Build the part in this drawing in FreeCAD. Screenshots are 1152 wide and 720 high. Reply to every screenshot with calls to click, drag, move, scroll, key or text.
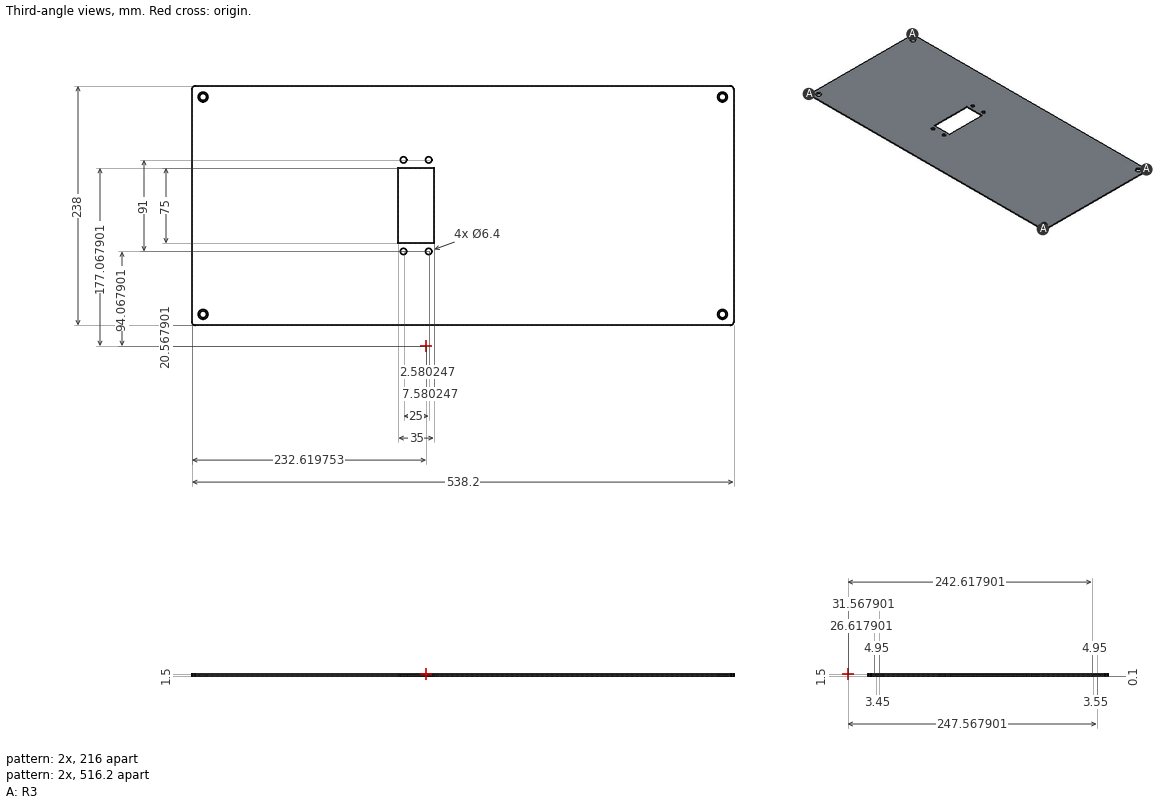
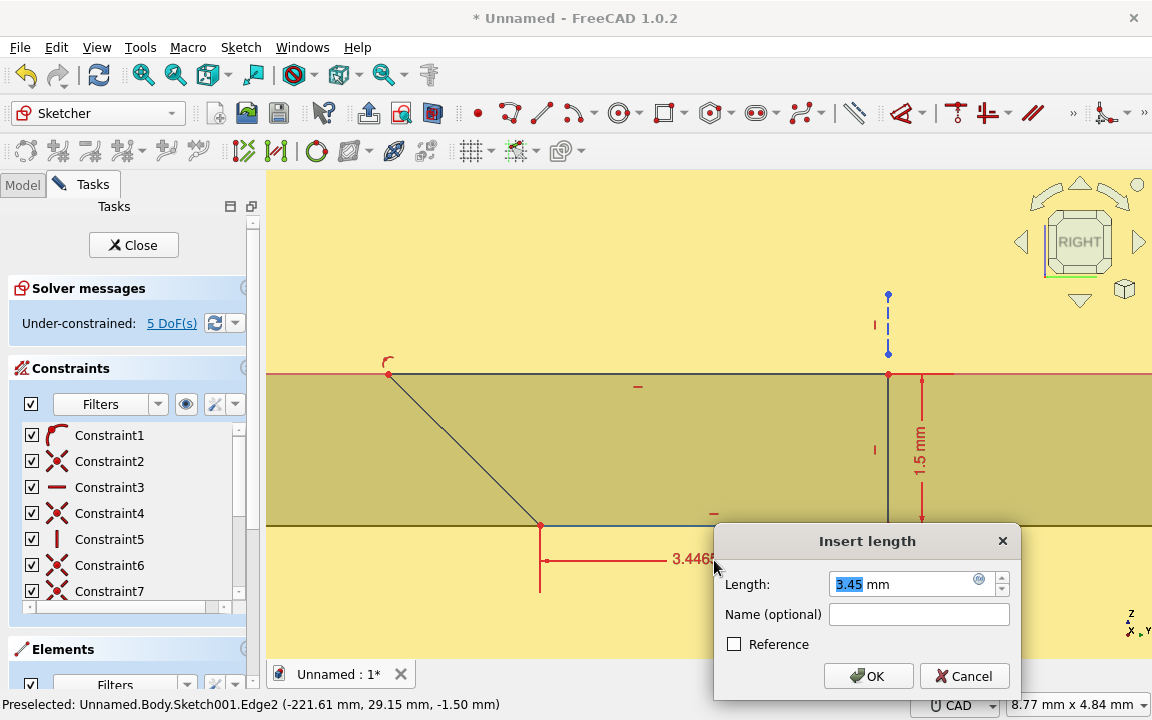
text(3.45)
key(Return)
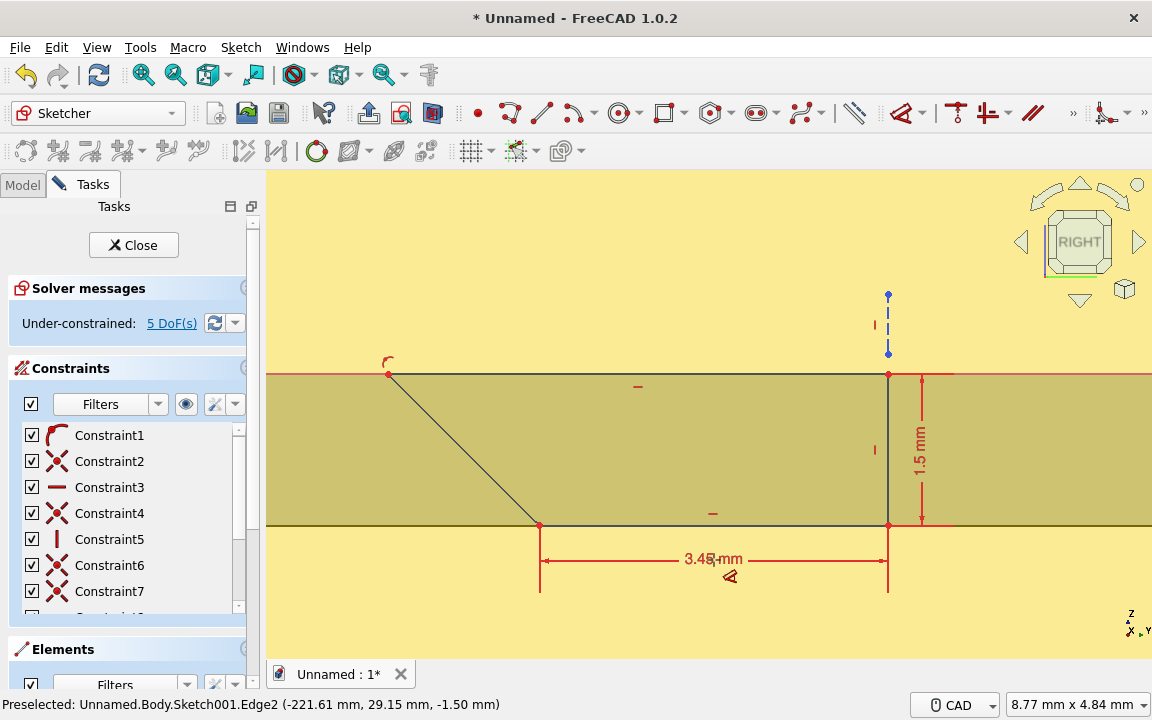
click(738, 374)
click(638, 340)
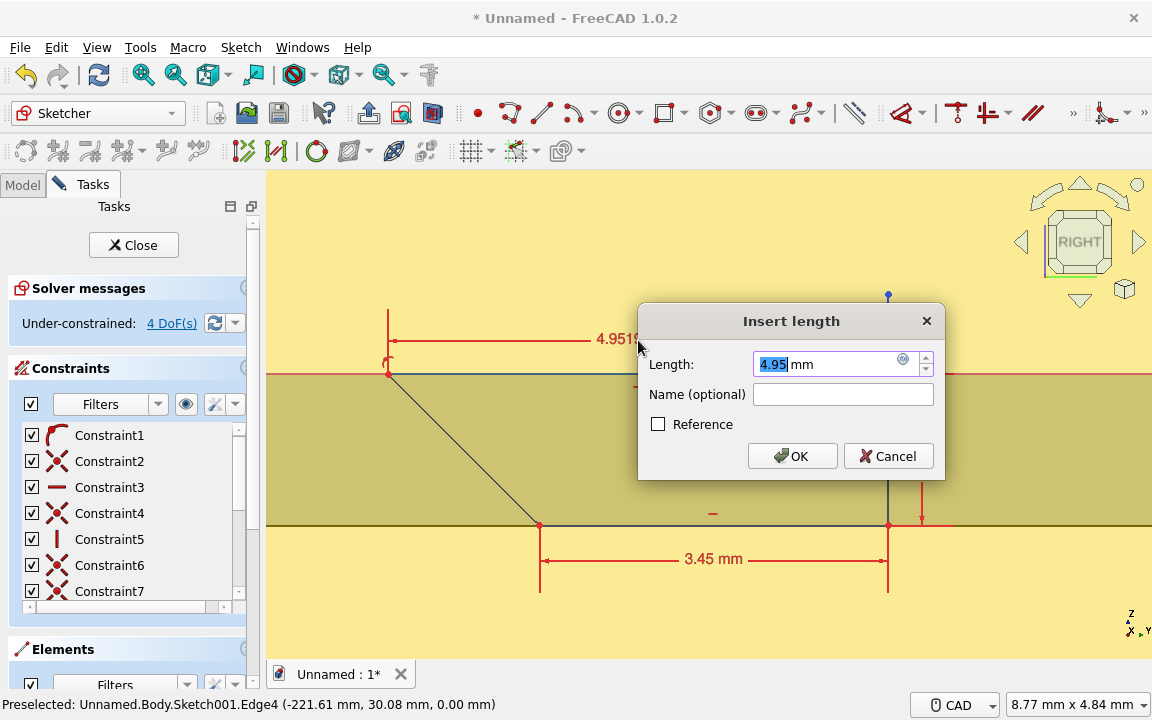
text(4.95)
key(Return)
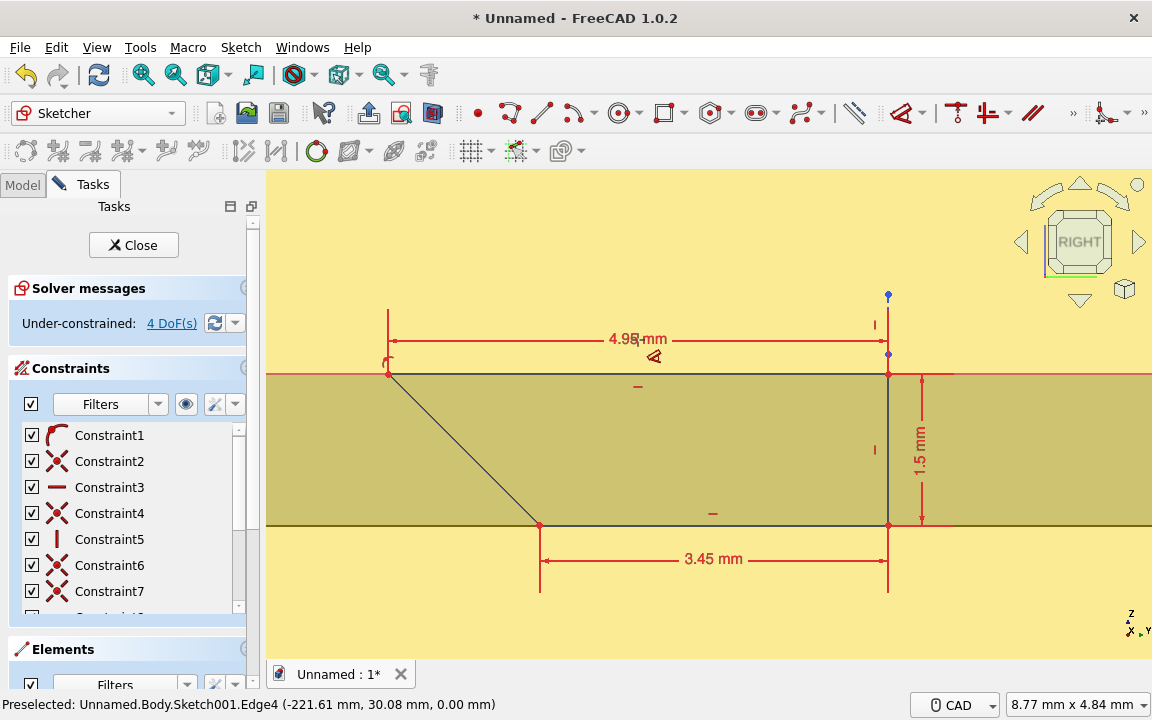
click(388, 374)
click(341, 340)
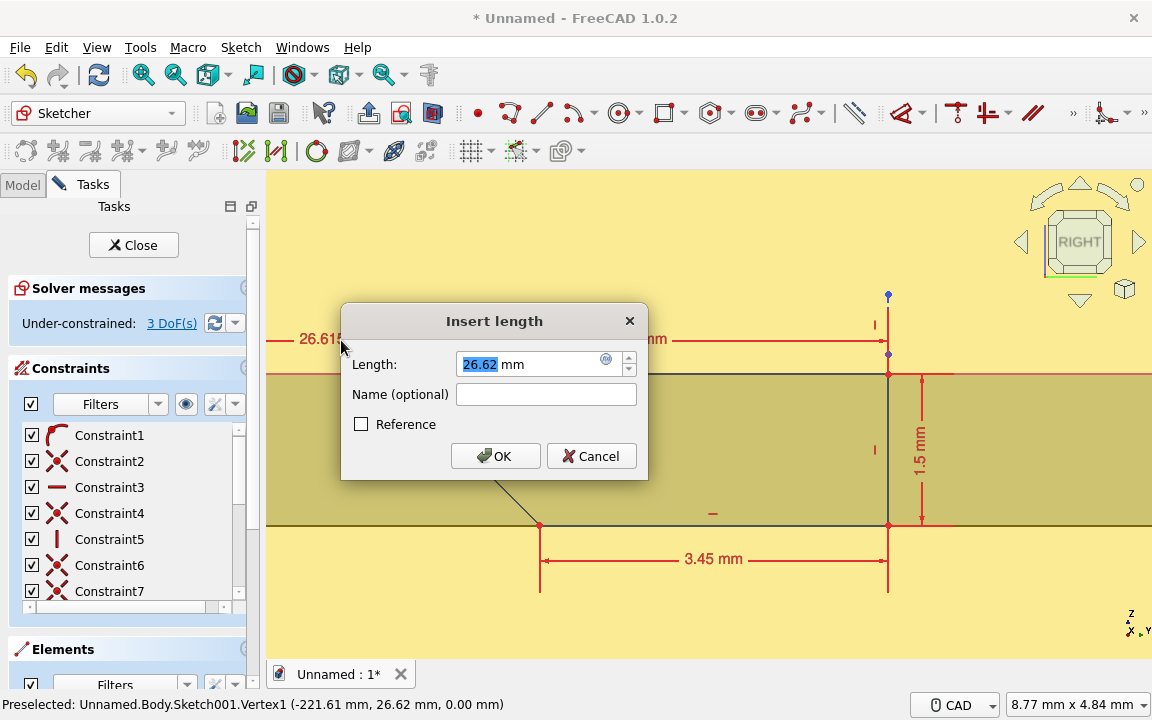
text(26.617901)
key(Return)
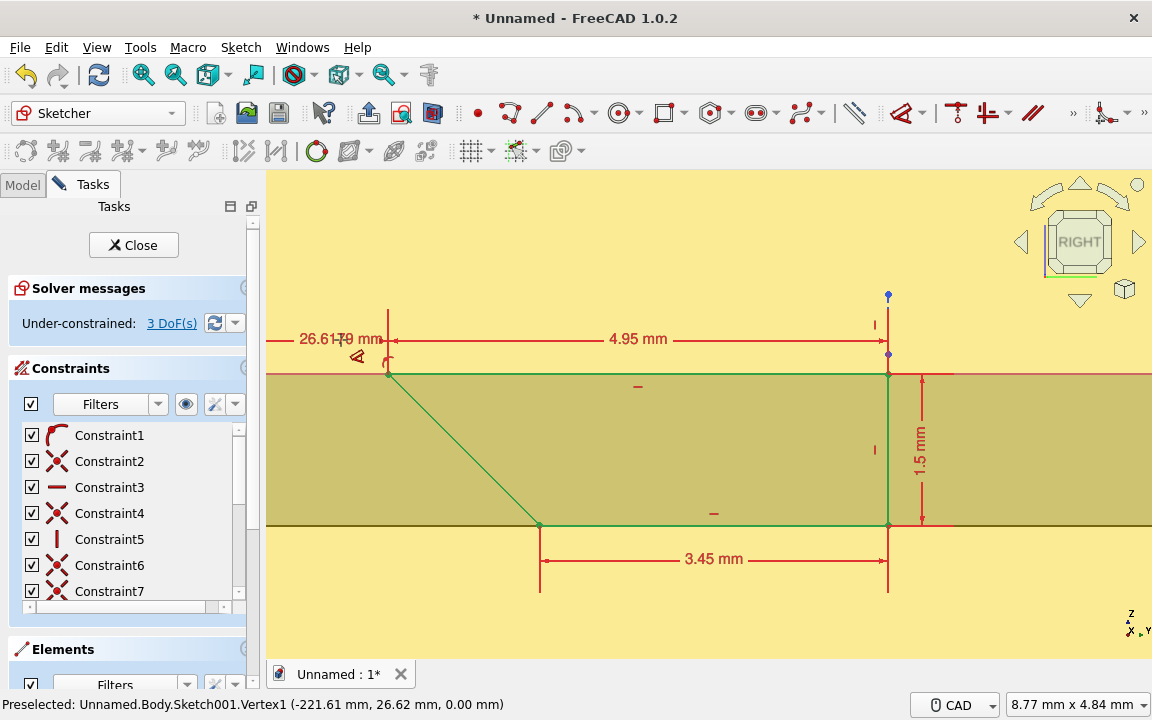
click(888, 355)
click(454, 321)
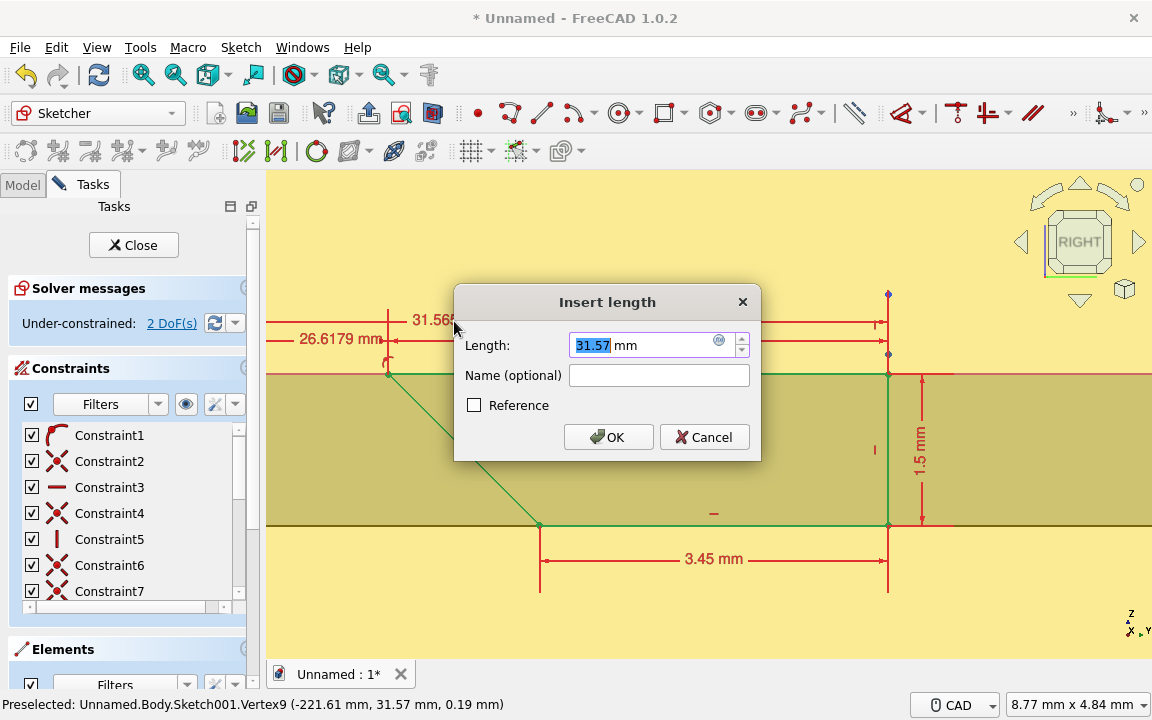
text(31.567901)
key(Return)
key(Escape)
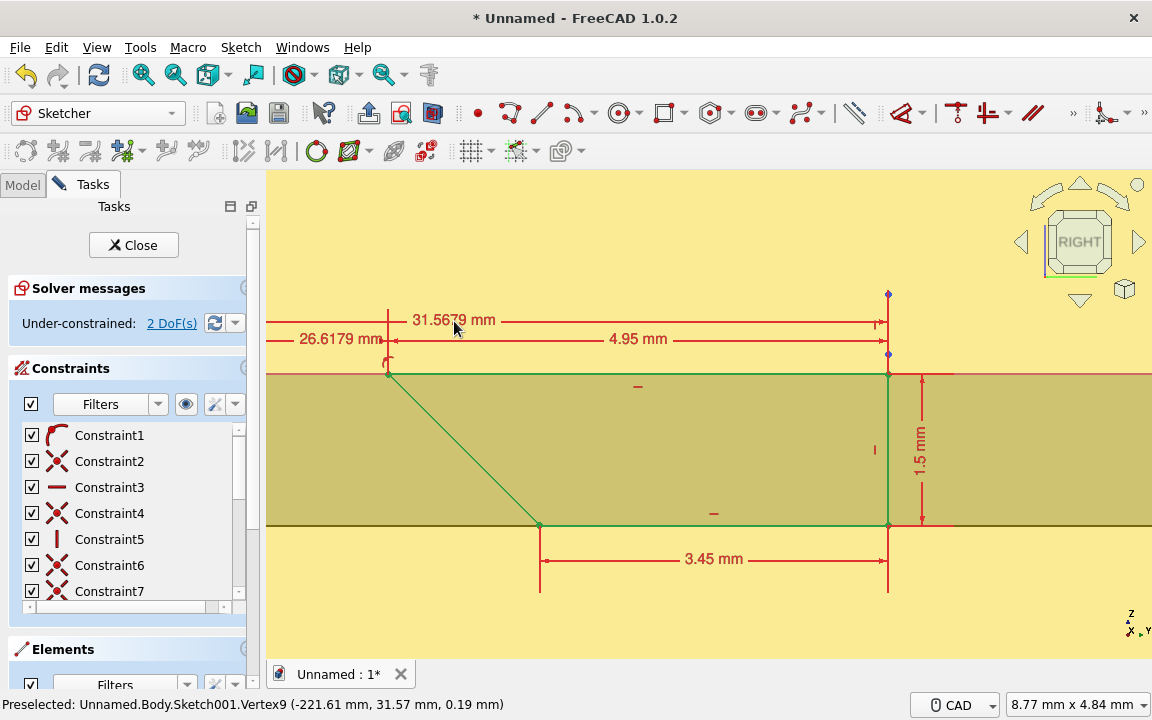
click(134, 245)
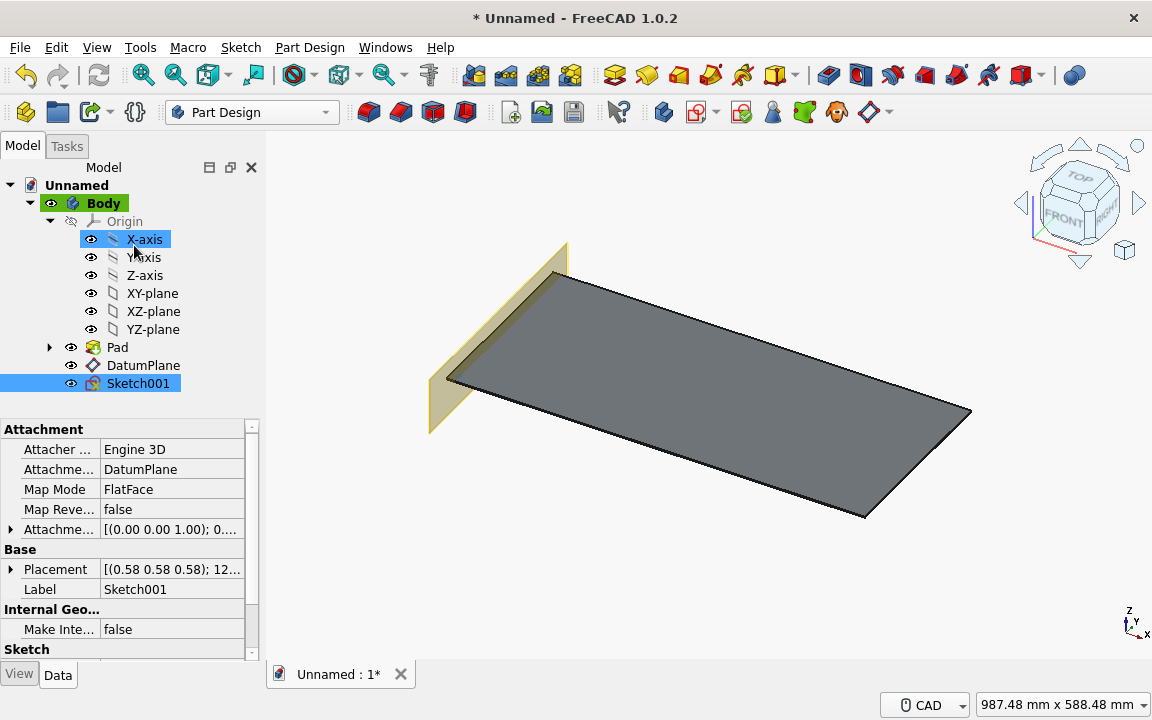
click(894, 76)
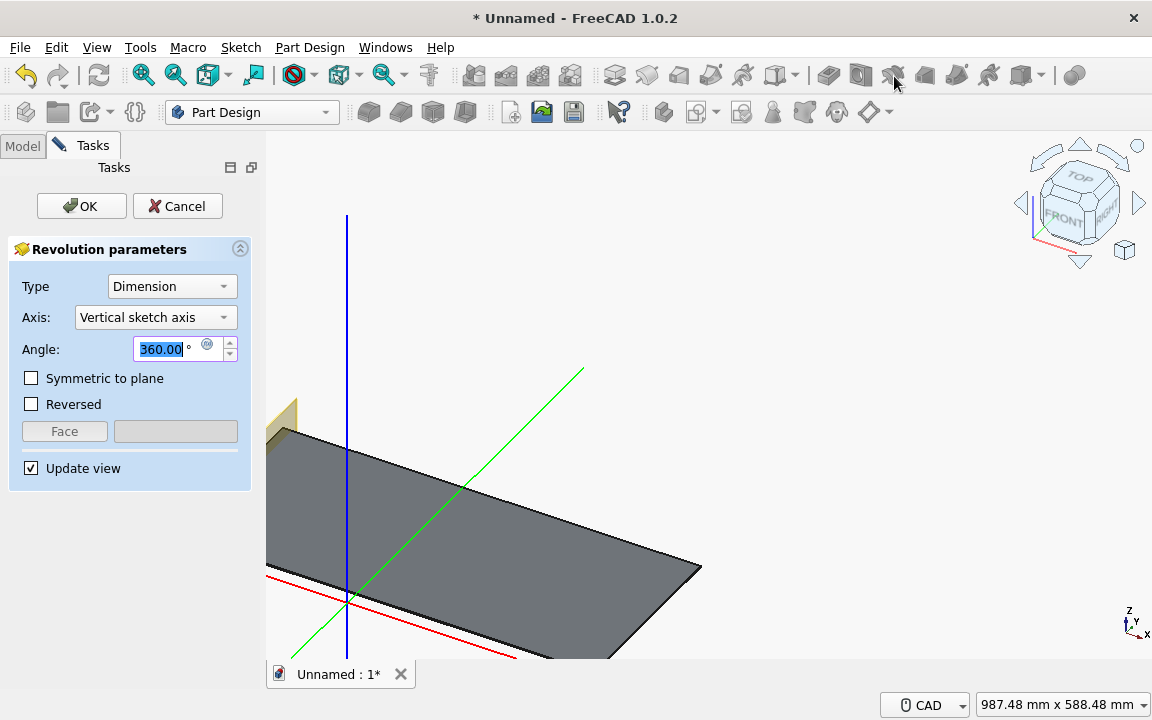
click(156, 318)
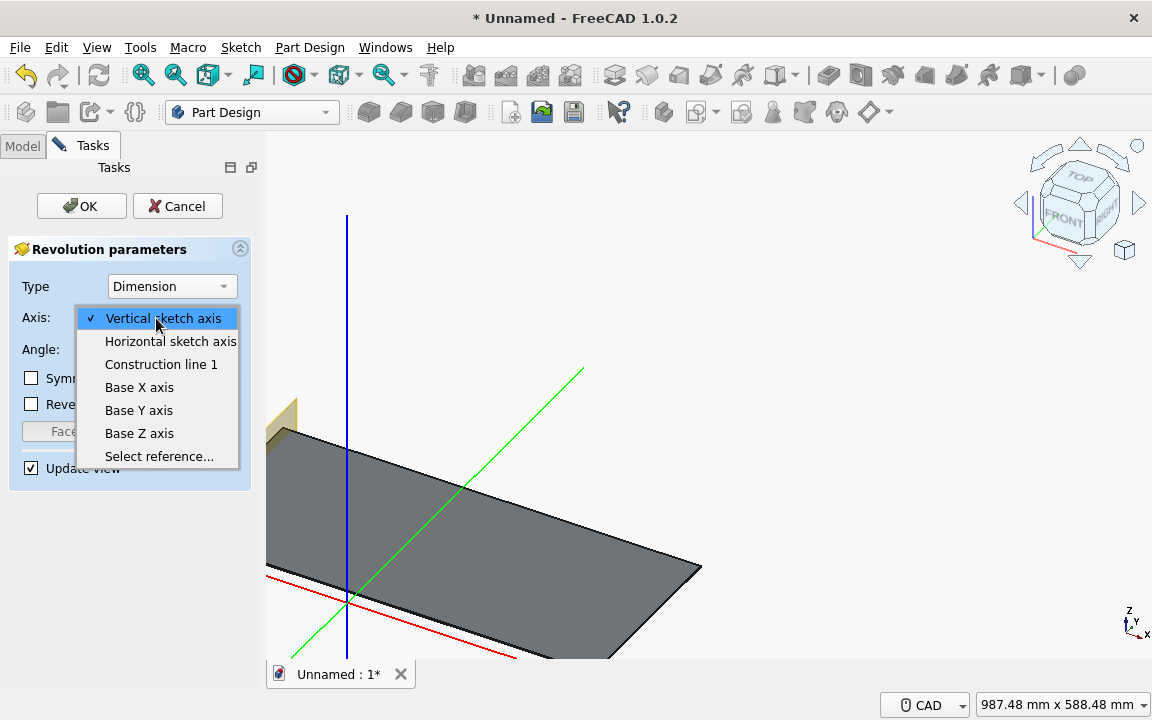
click(156, 364)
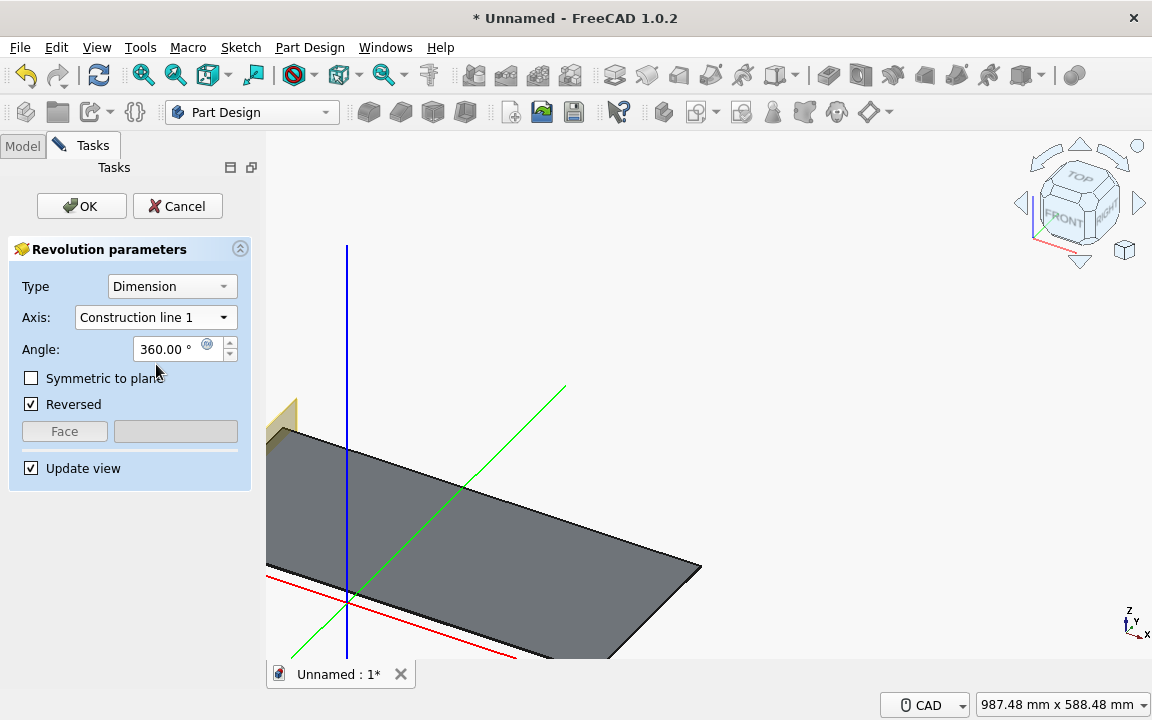
click(82, 206)